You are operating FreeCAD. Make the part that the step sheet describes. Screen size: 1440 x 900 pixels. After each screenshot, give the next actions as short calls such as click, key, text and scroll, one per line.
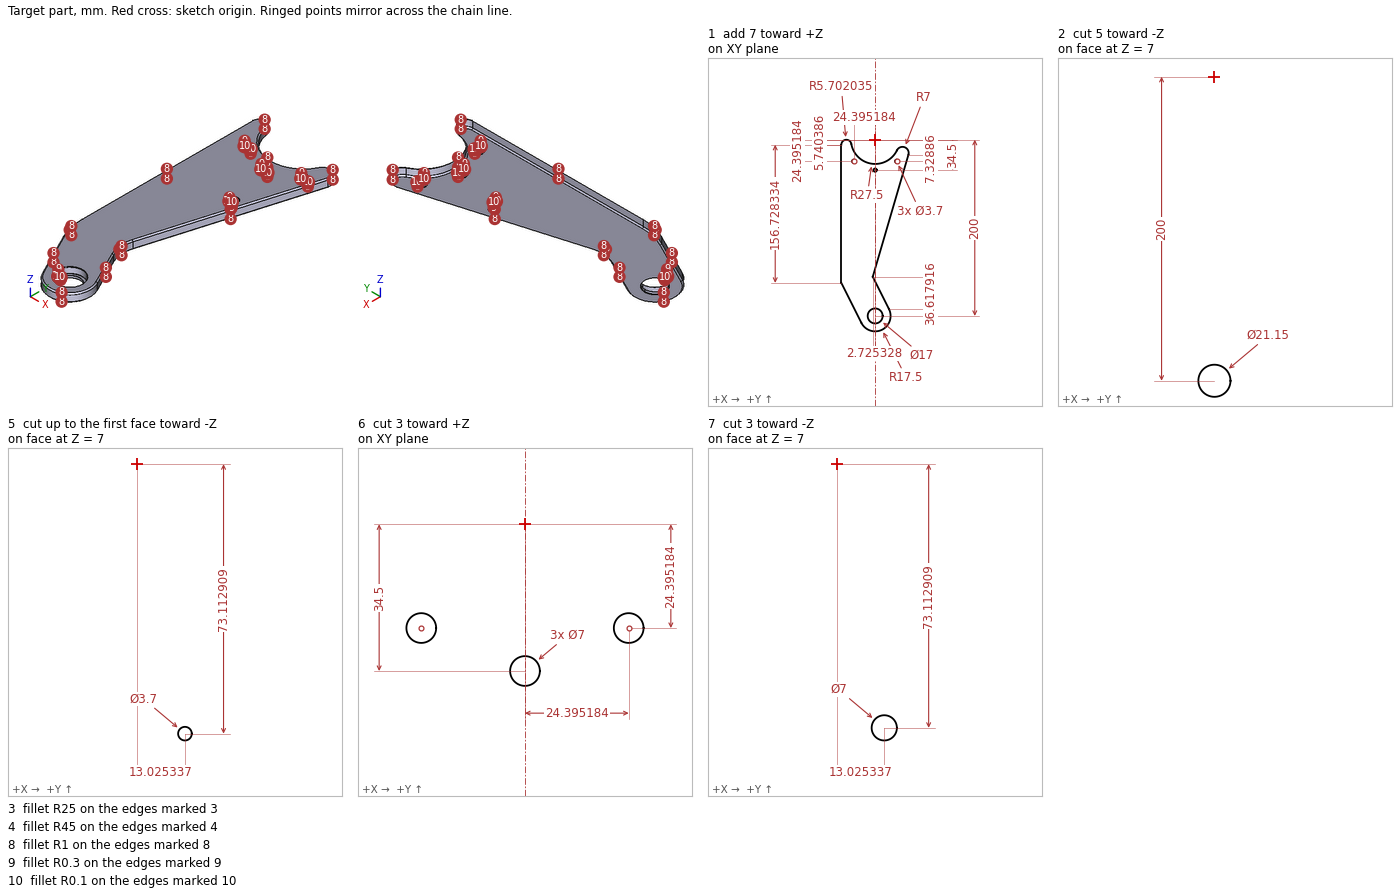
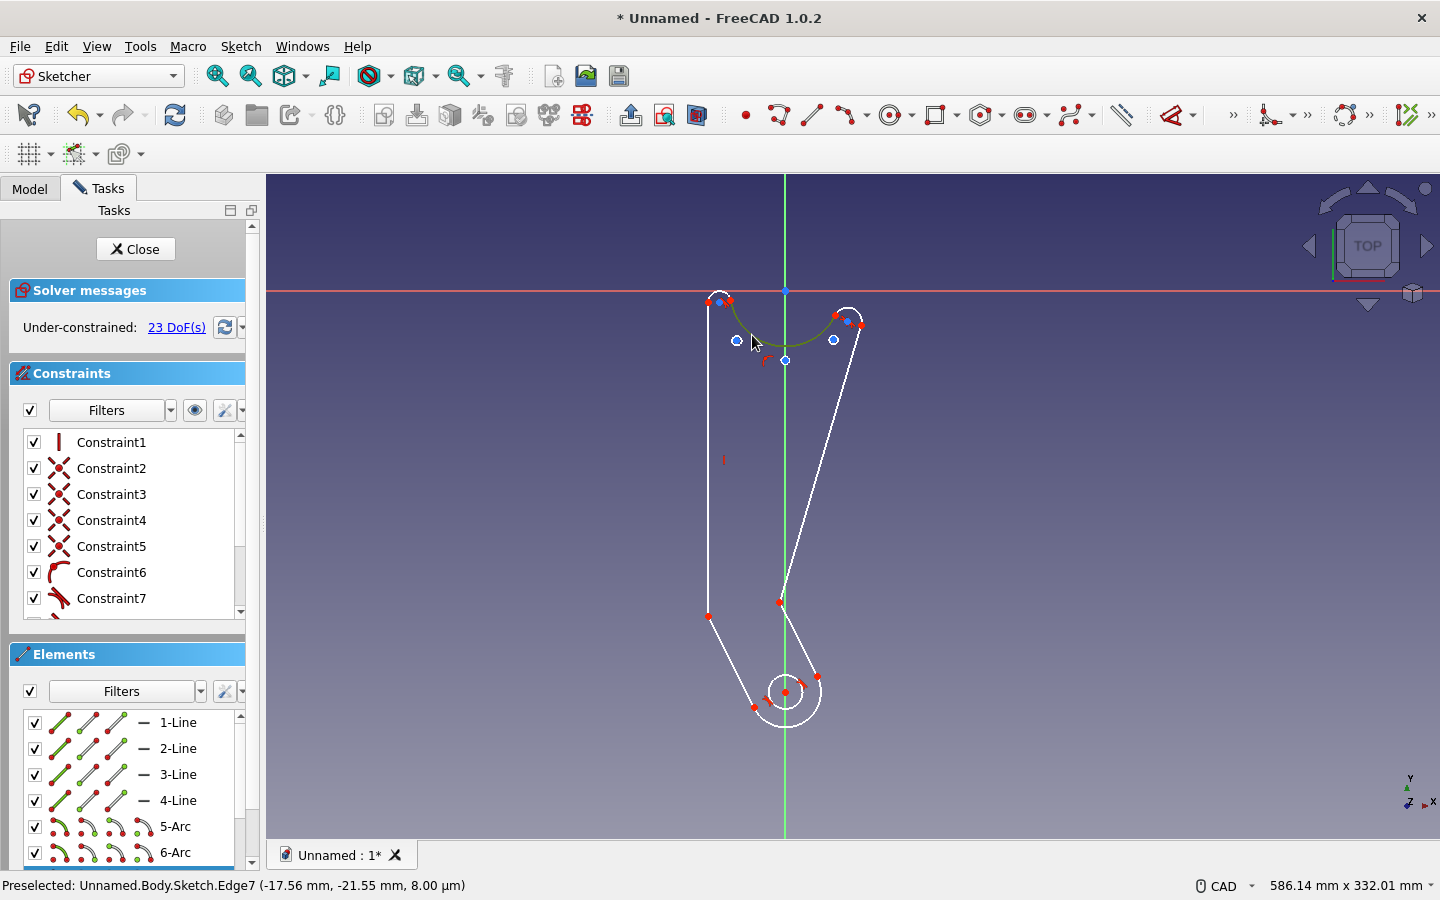
scroll(725, 293, up, 2)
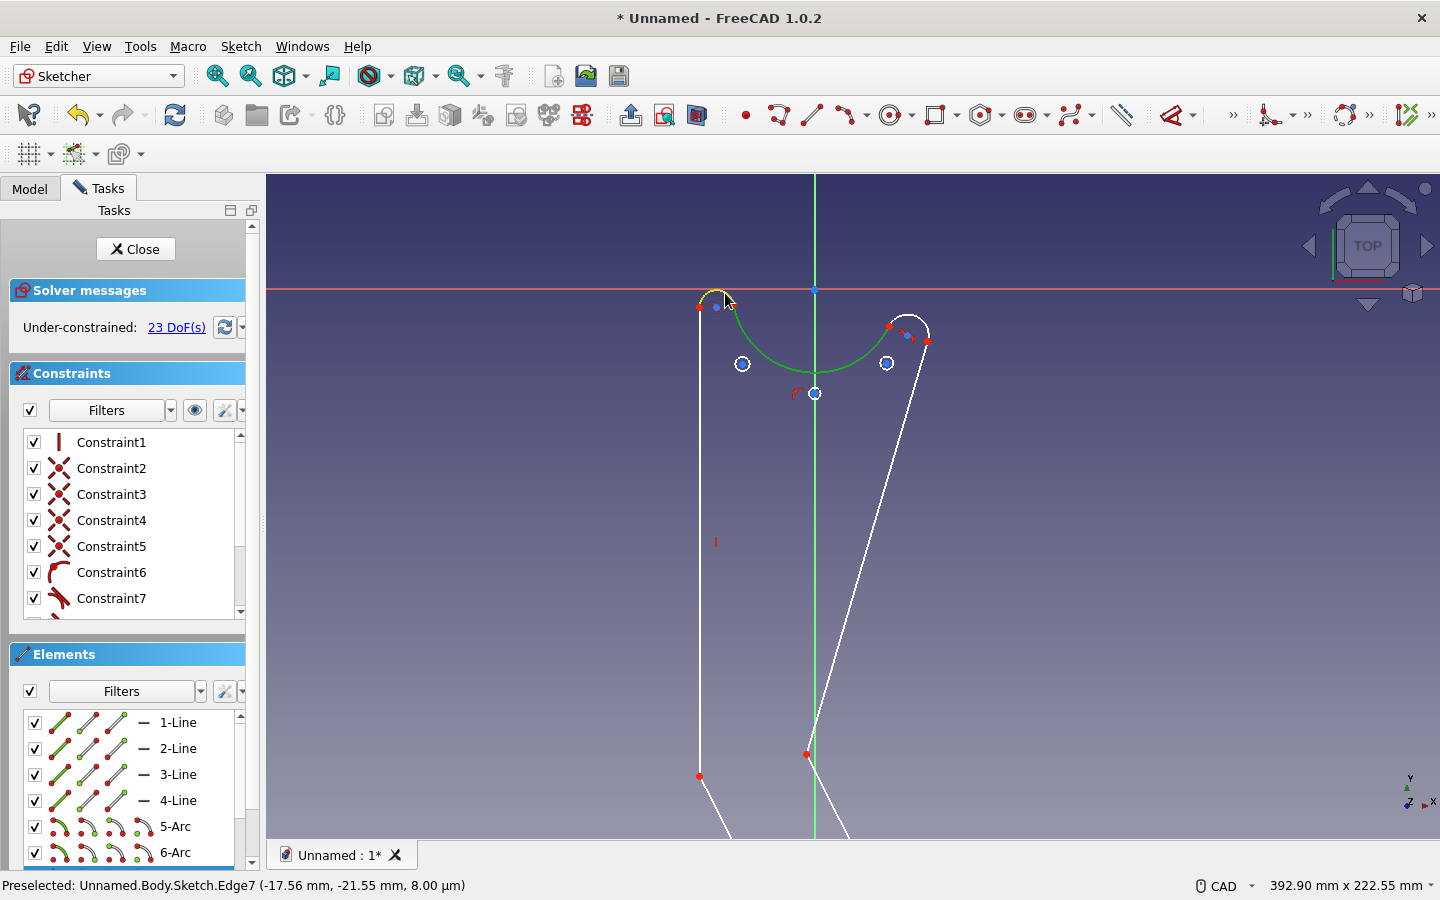
click(725, 292)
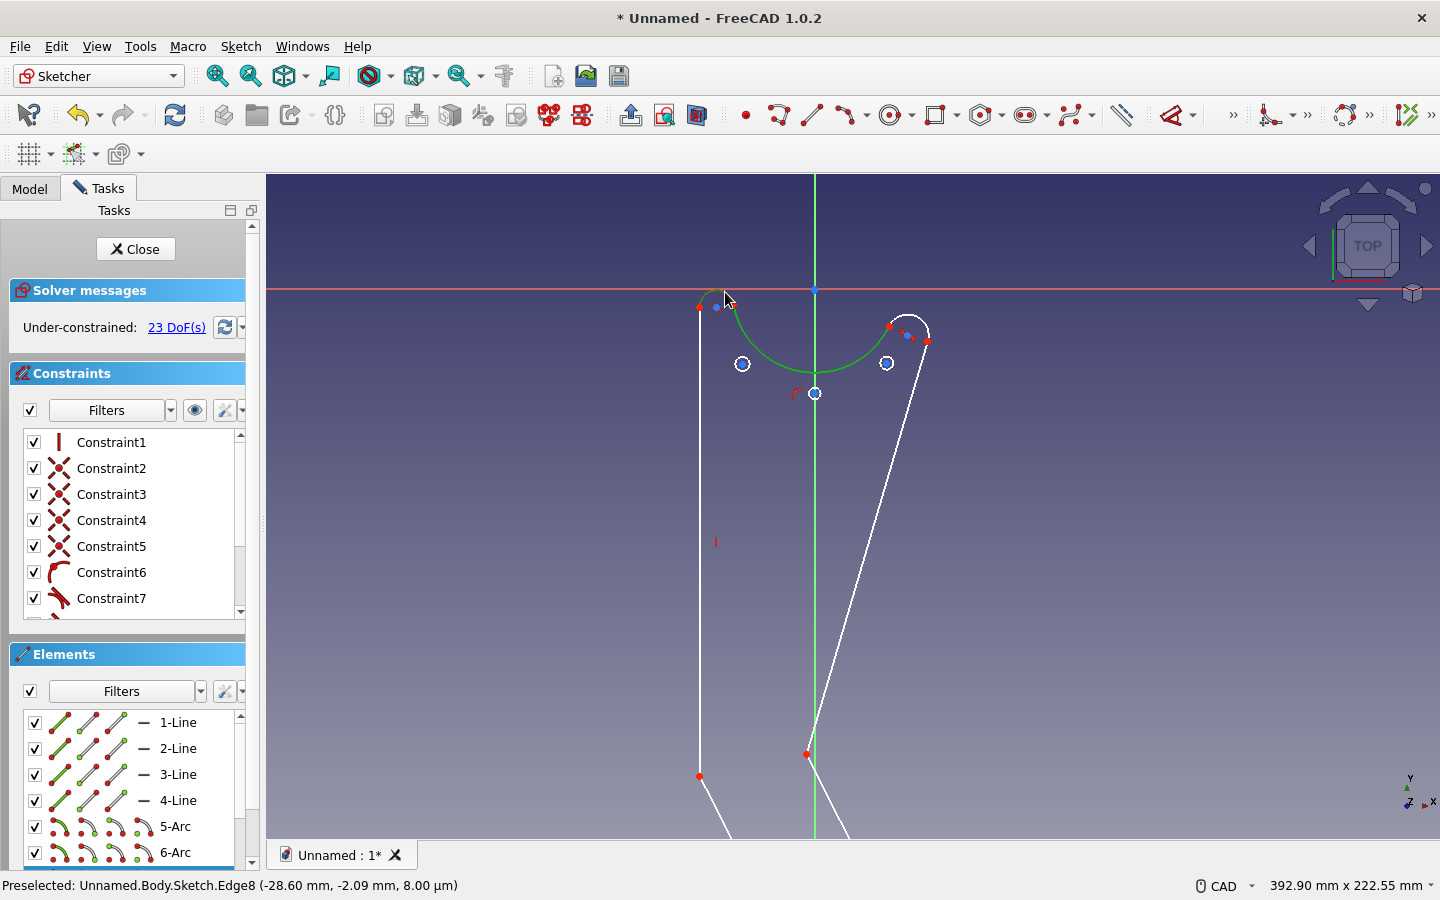
key(t)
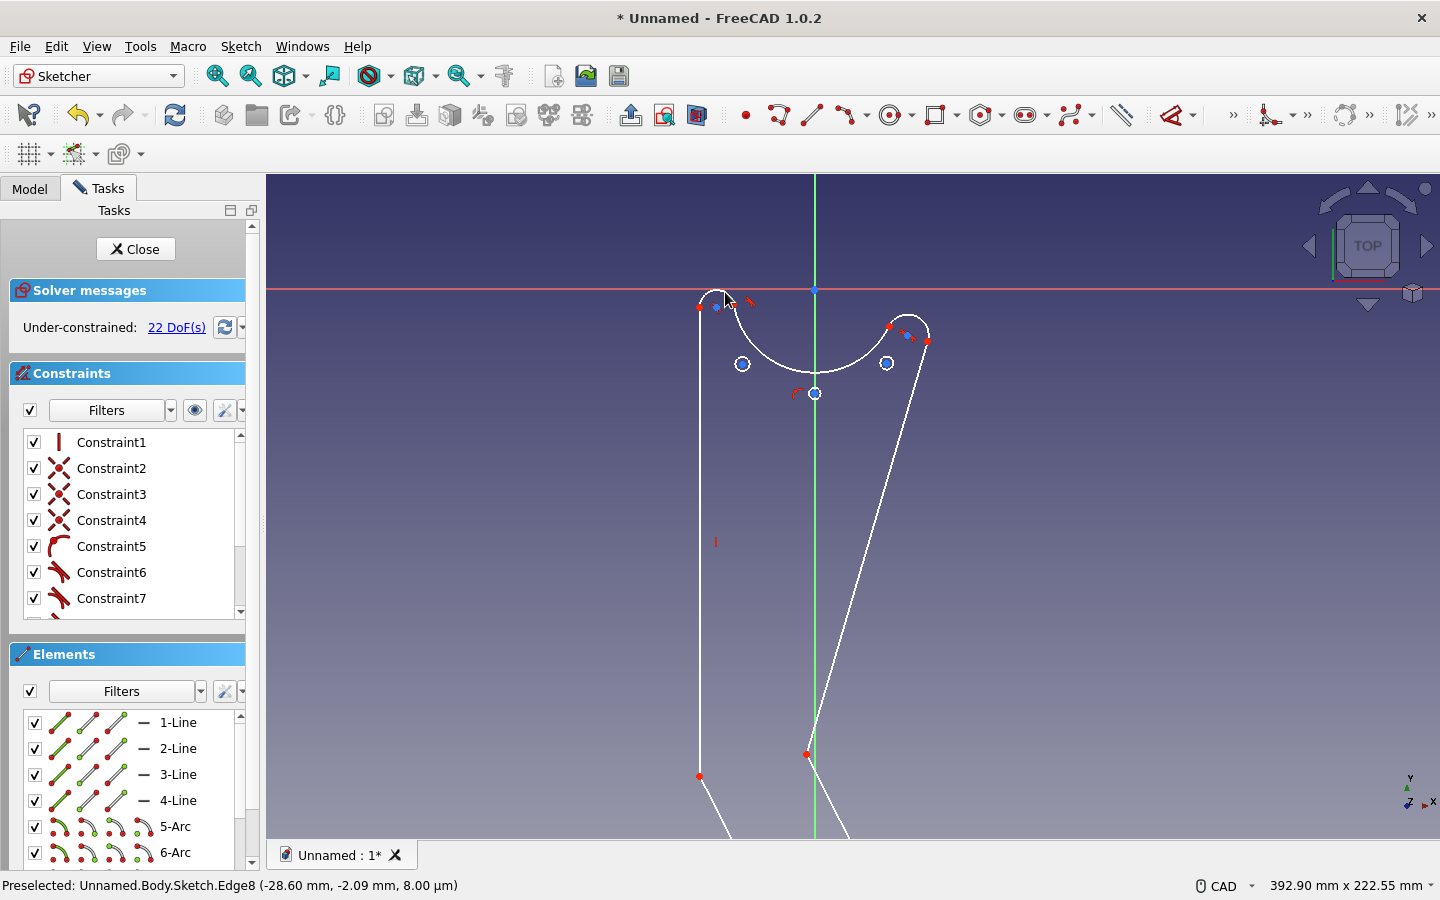
scroll(815, 290, up, 10)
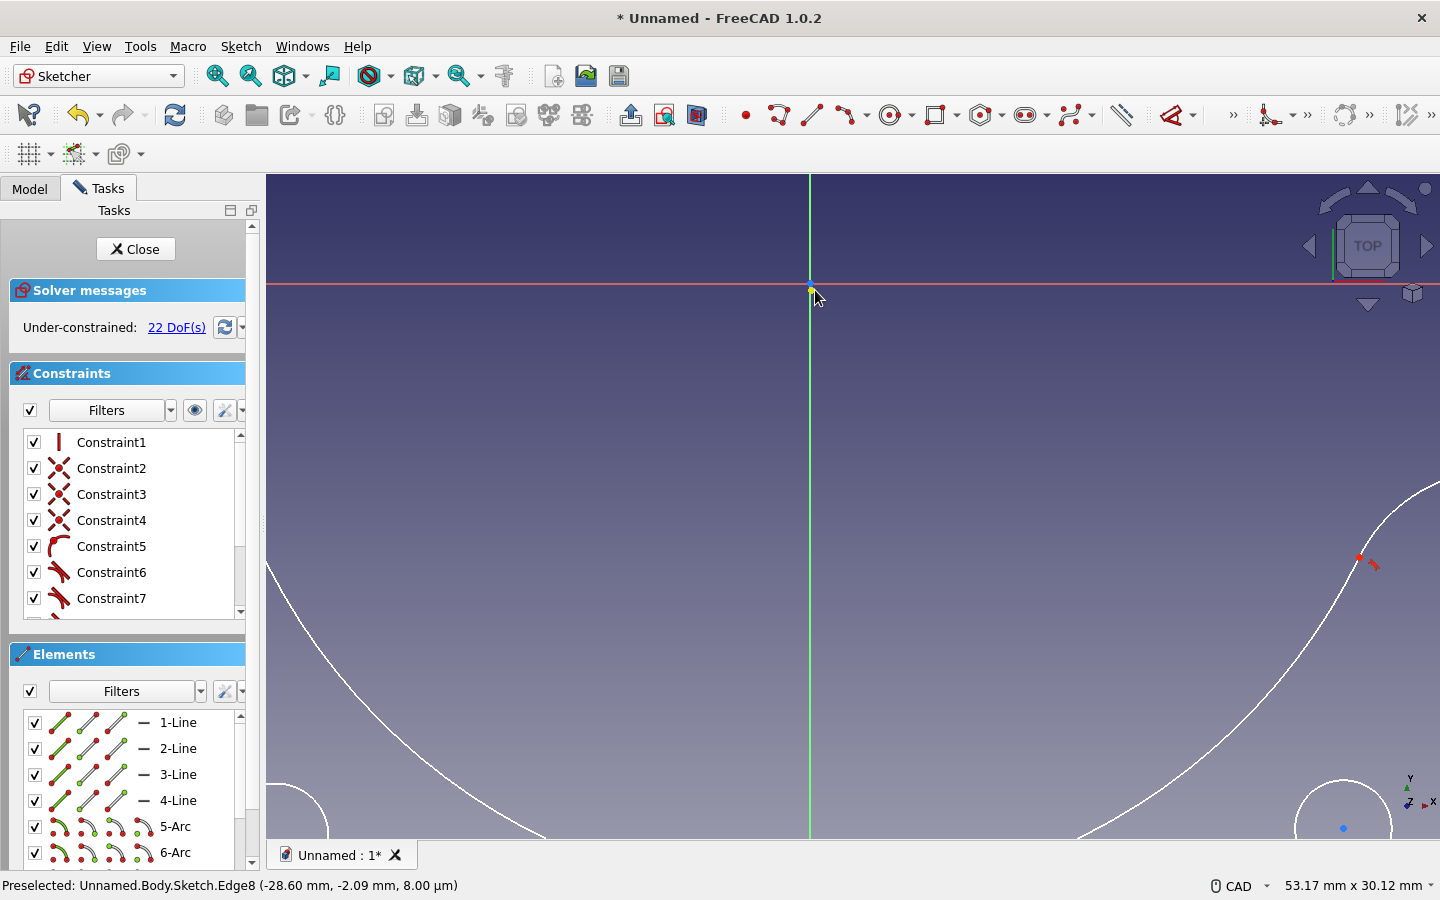
drag(800, 274, 822, 300)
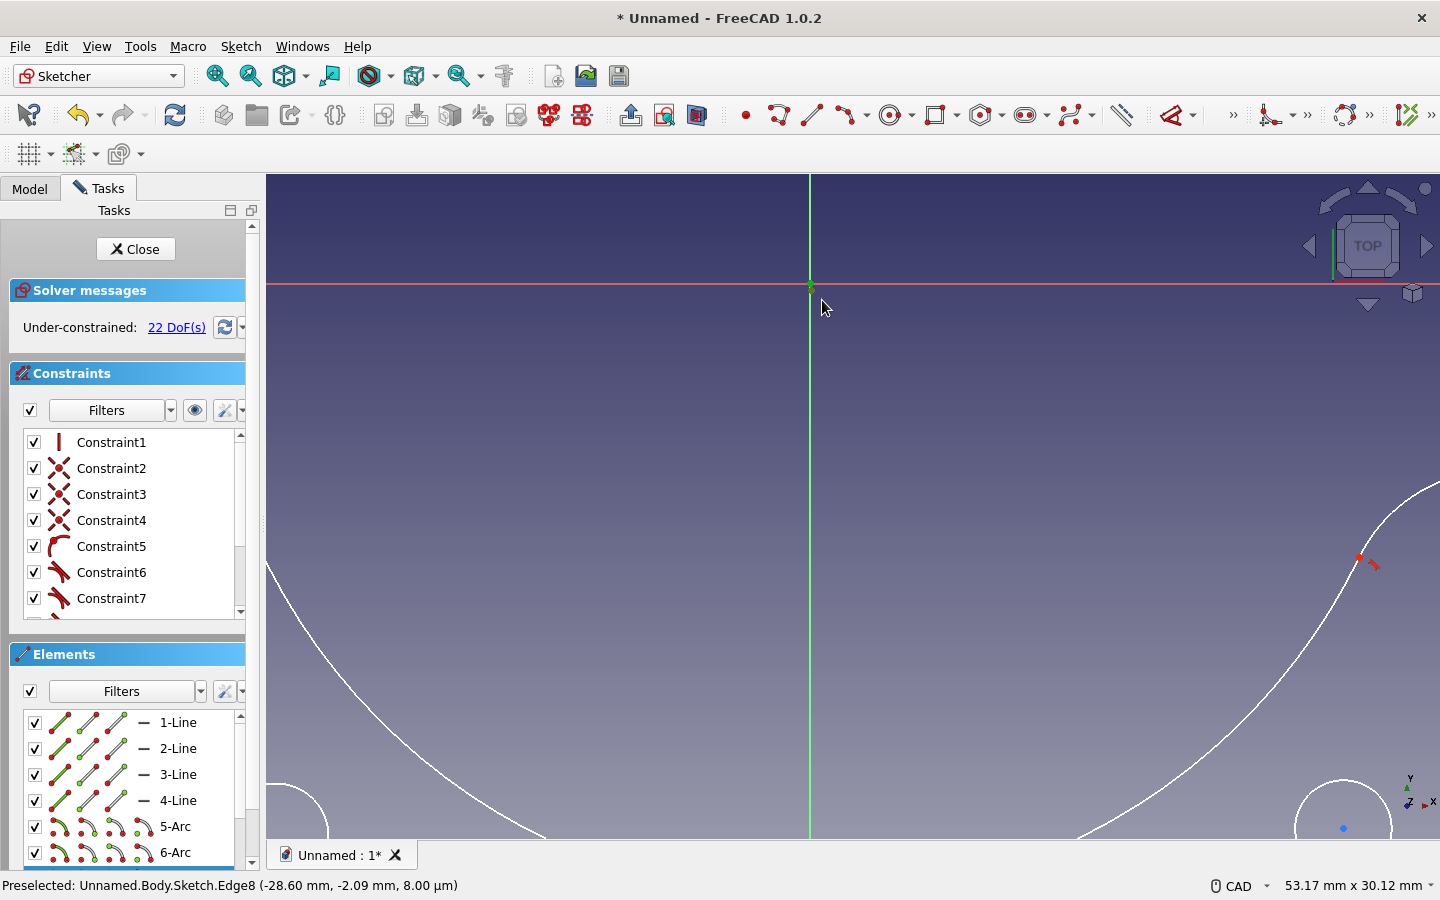
key(c)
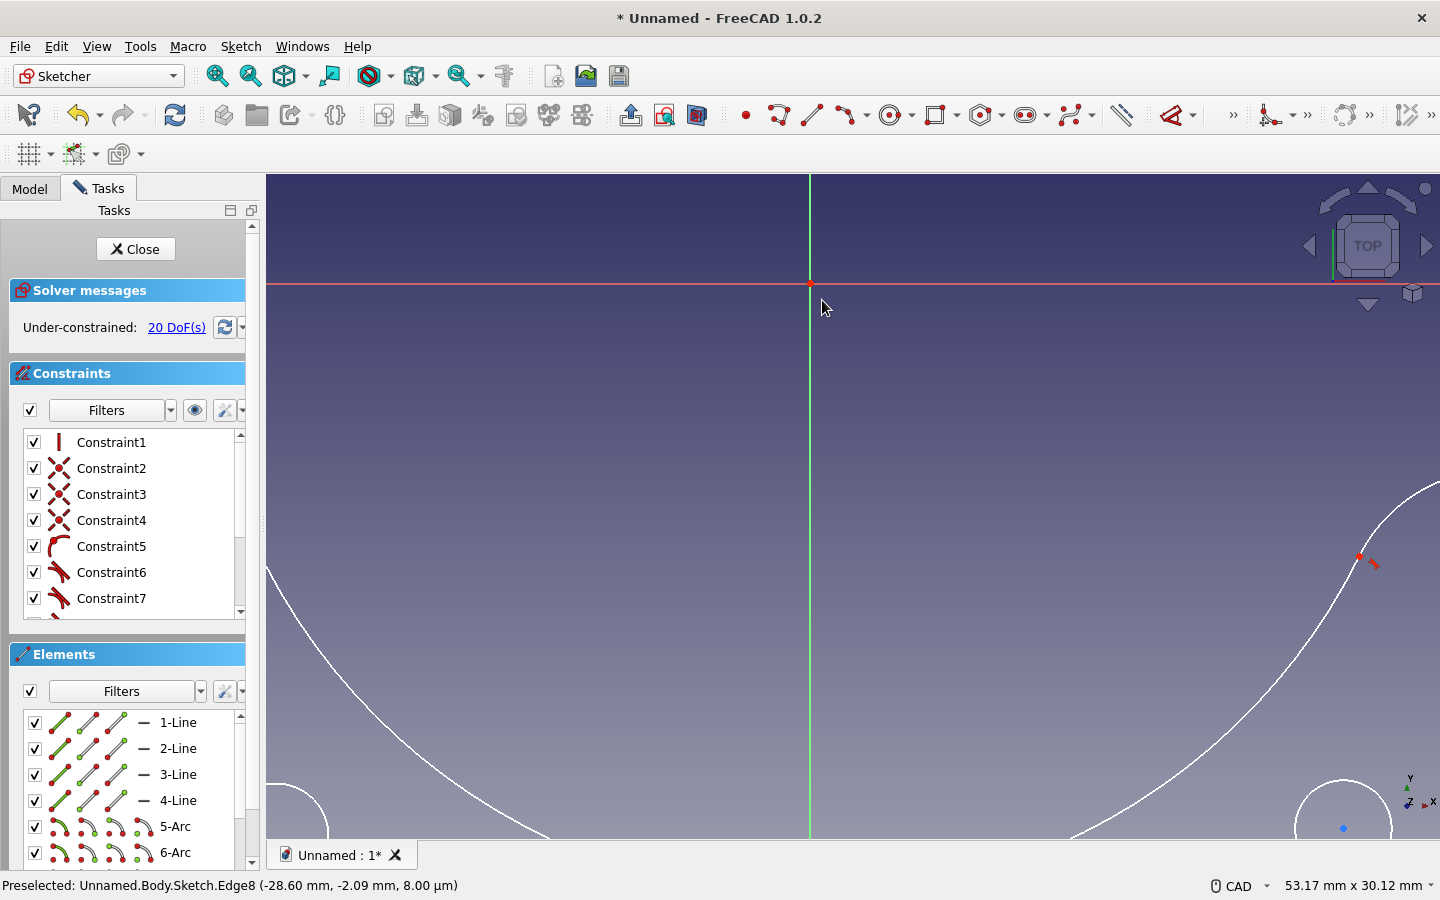
scroll(783, 291, down, 12)